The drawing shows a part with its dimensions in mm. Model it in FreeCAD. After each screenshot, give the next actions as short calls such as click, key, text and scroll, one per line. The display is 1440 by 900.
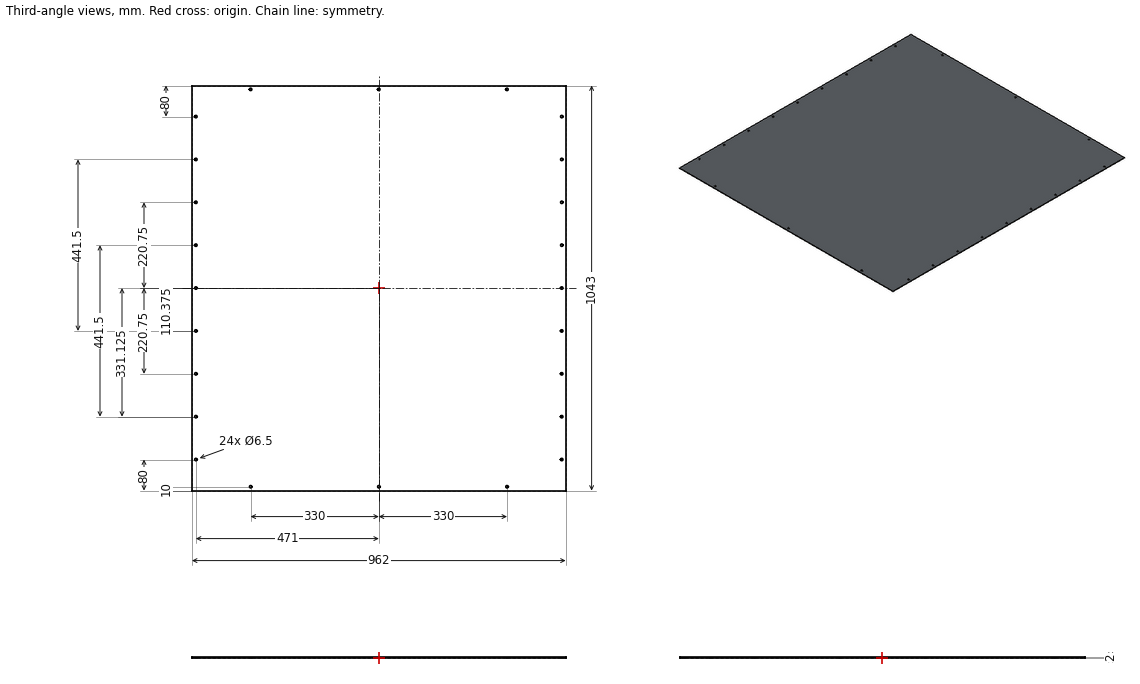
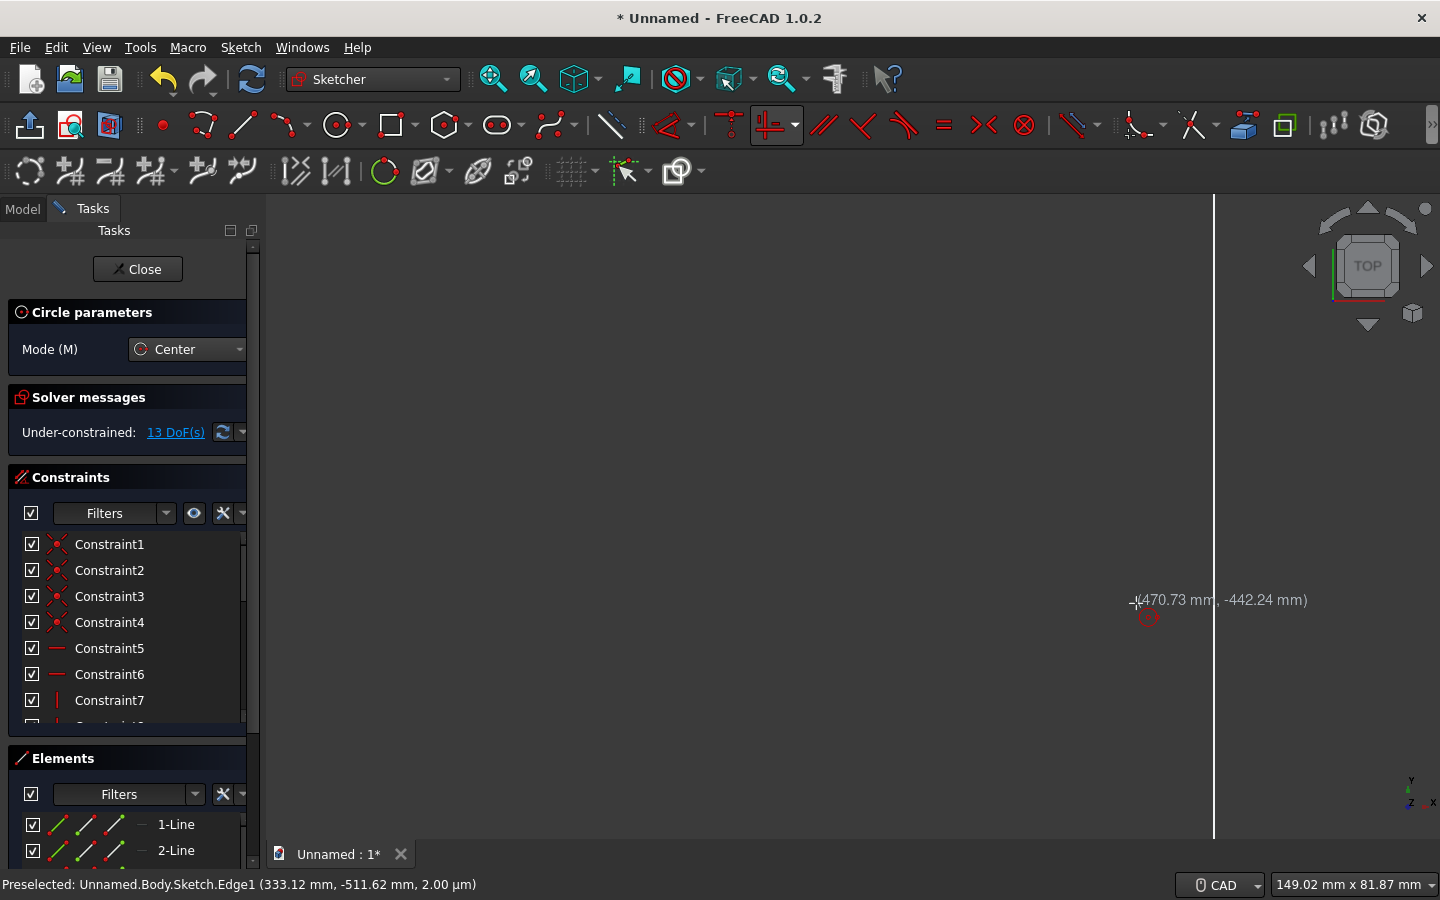
scroll(961, 694, down, 15)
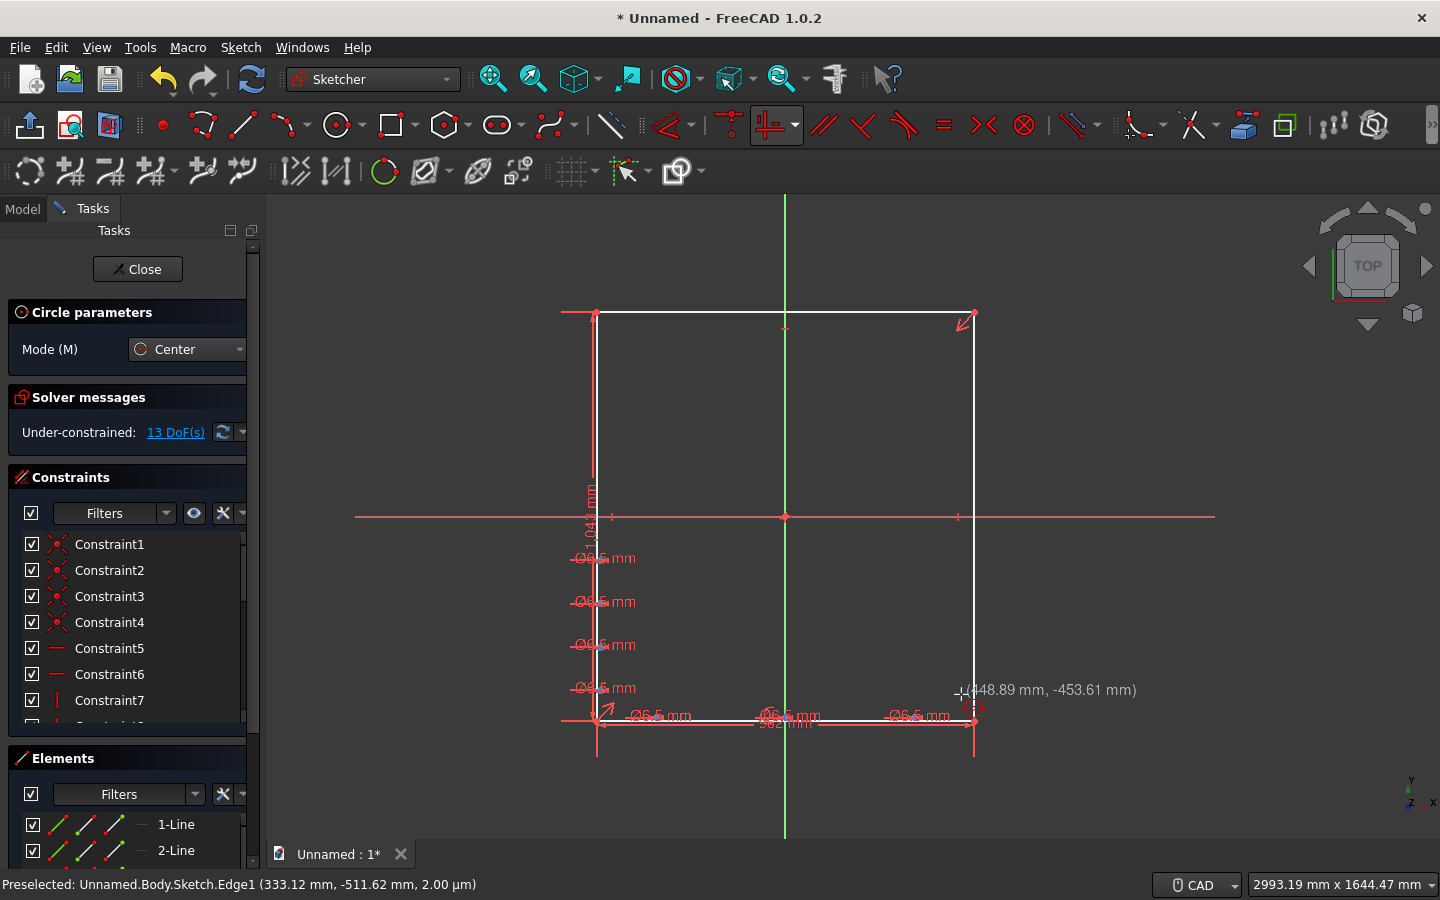
scroll(970, 690, up, 7)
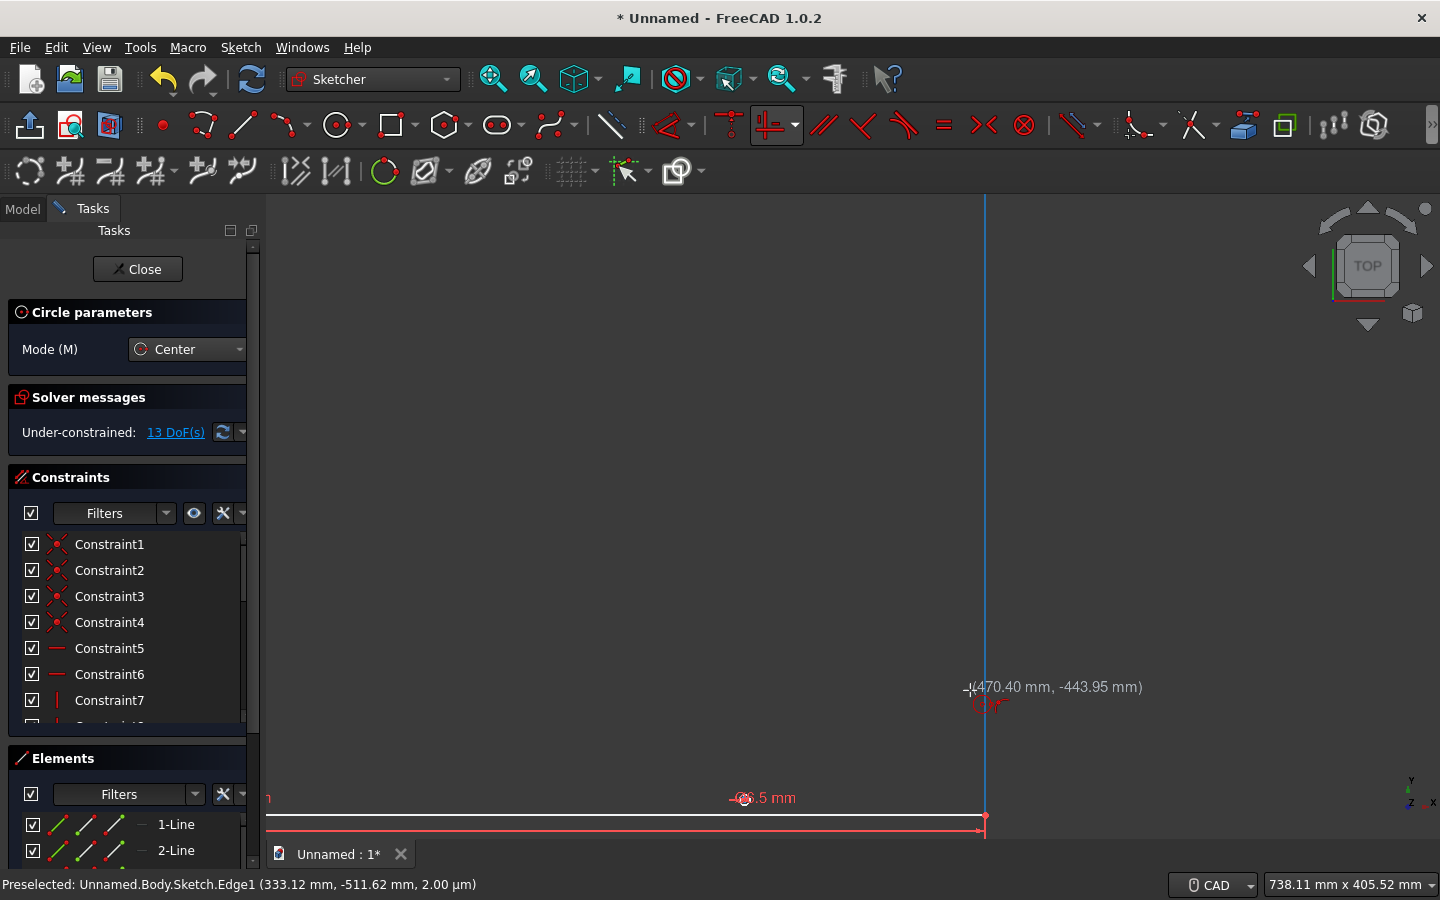
click(969, 688)
move(965, 684)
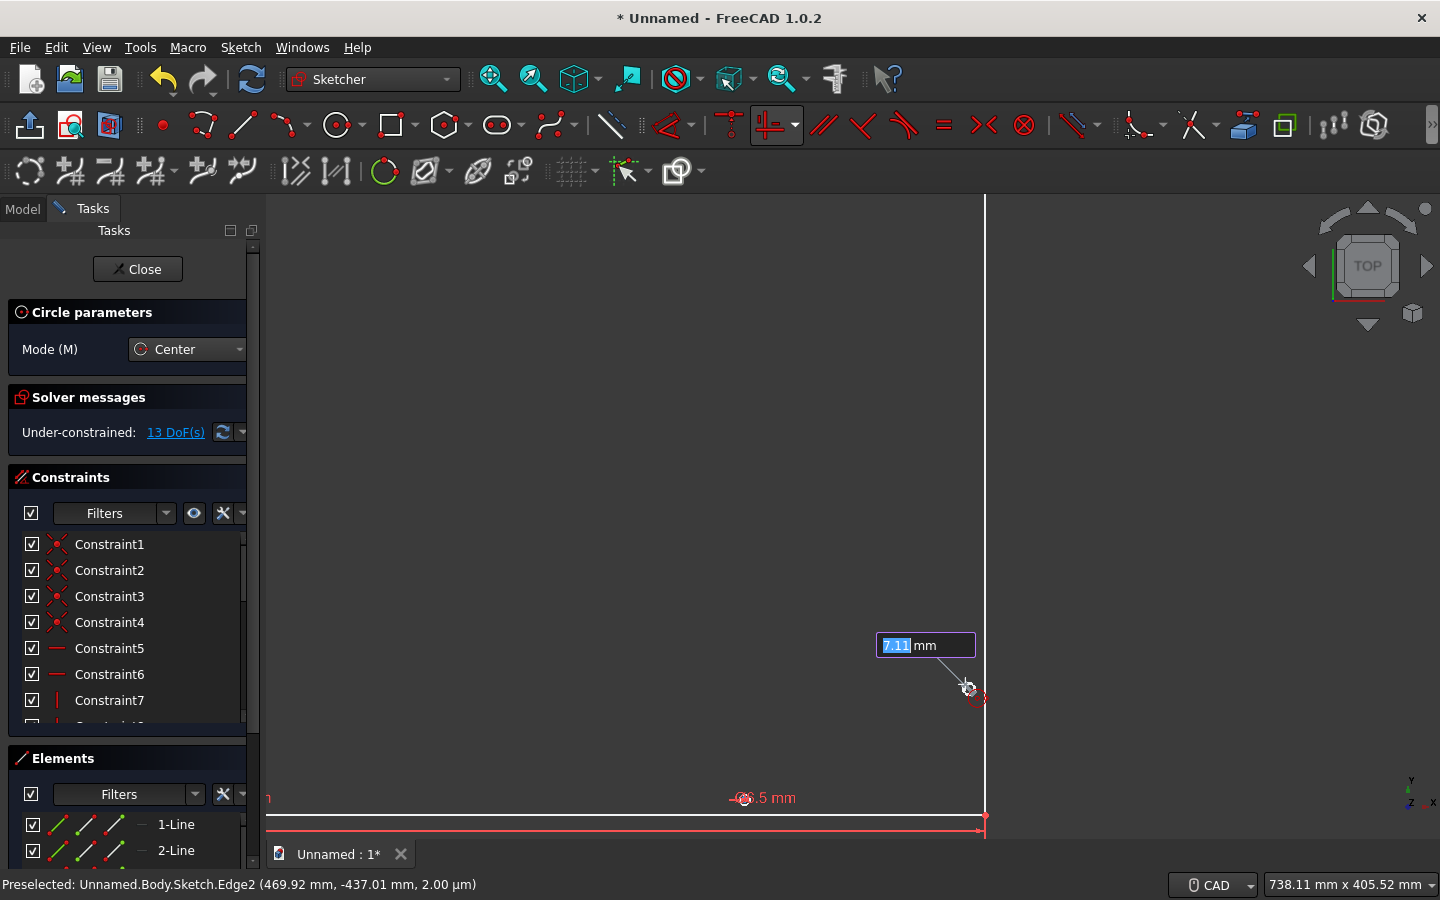
text(6.5)
key(Return)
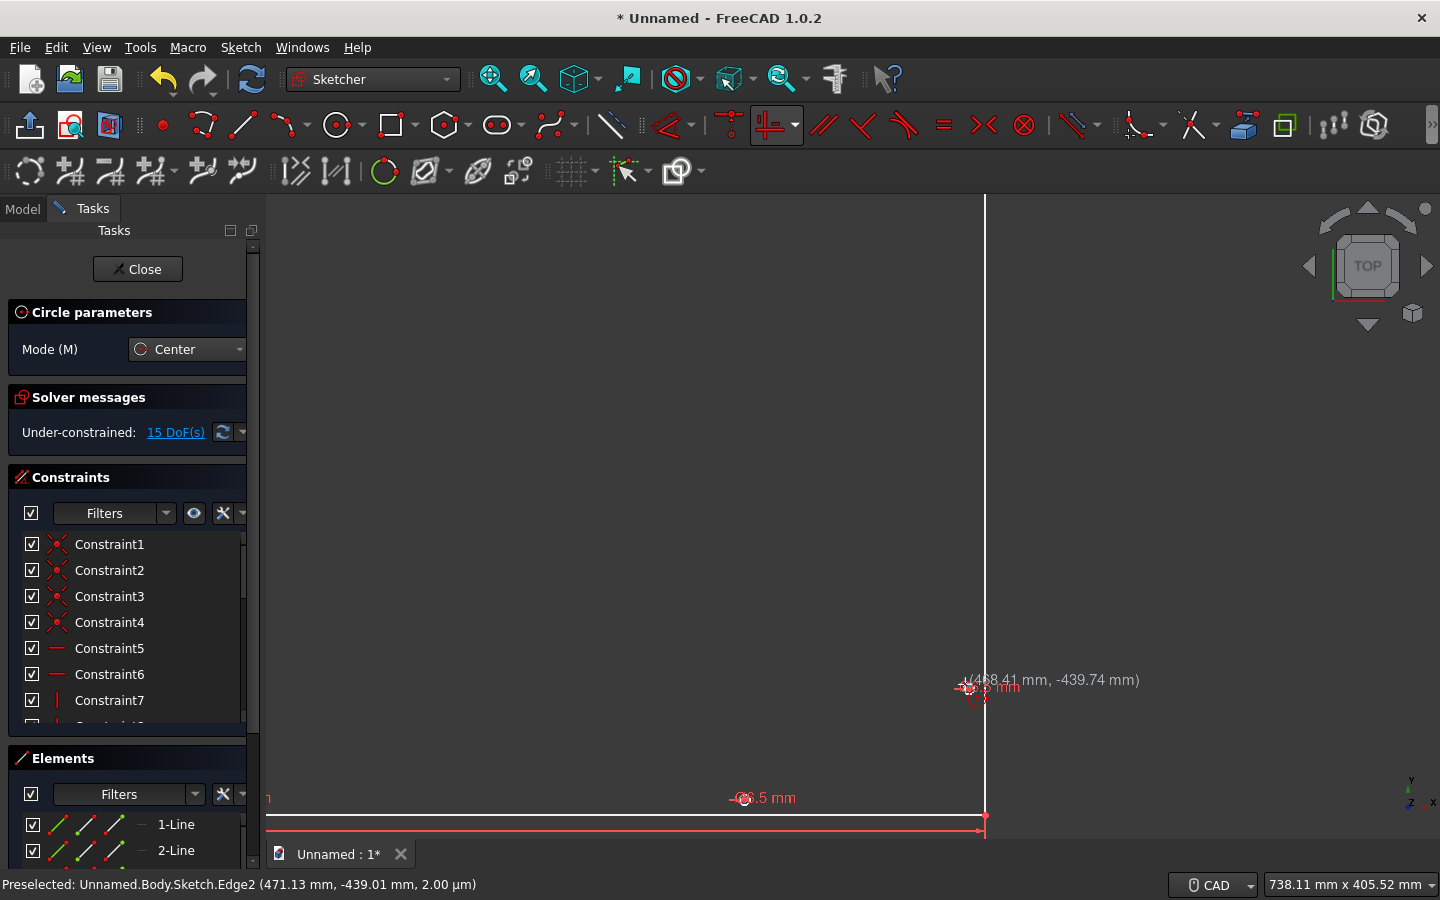
scroll(969, 512, up, 8)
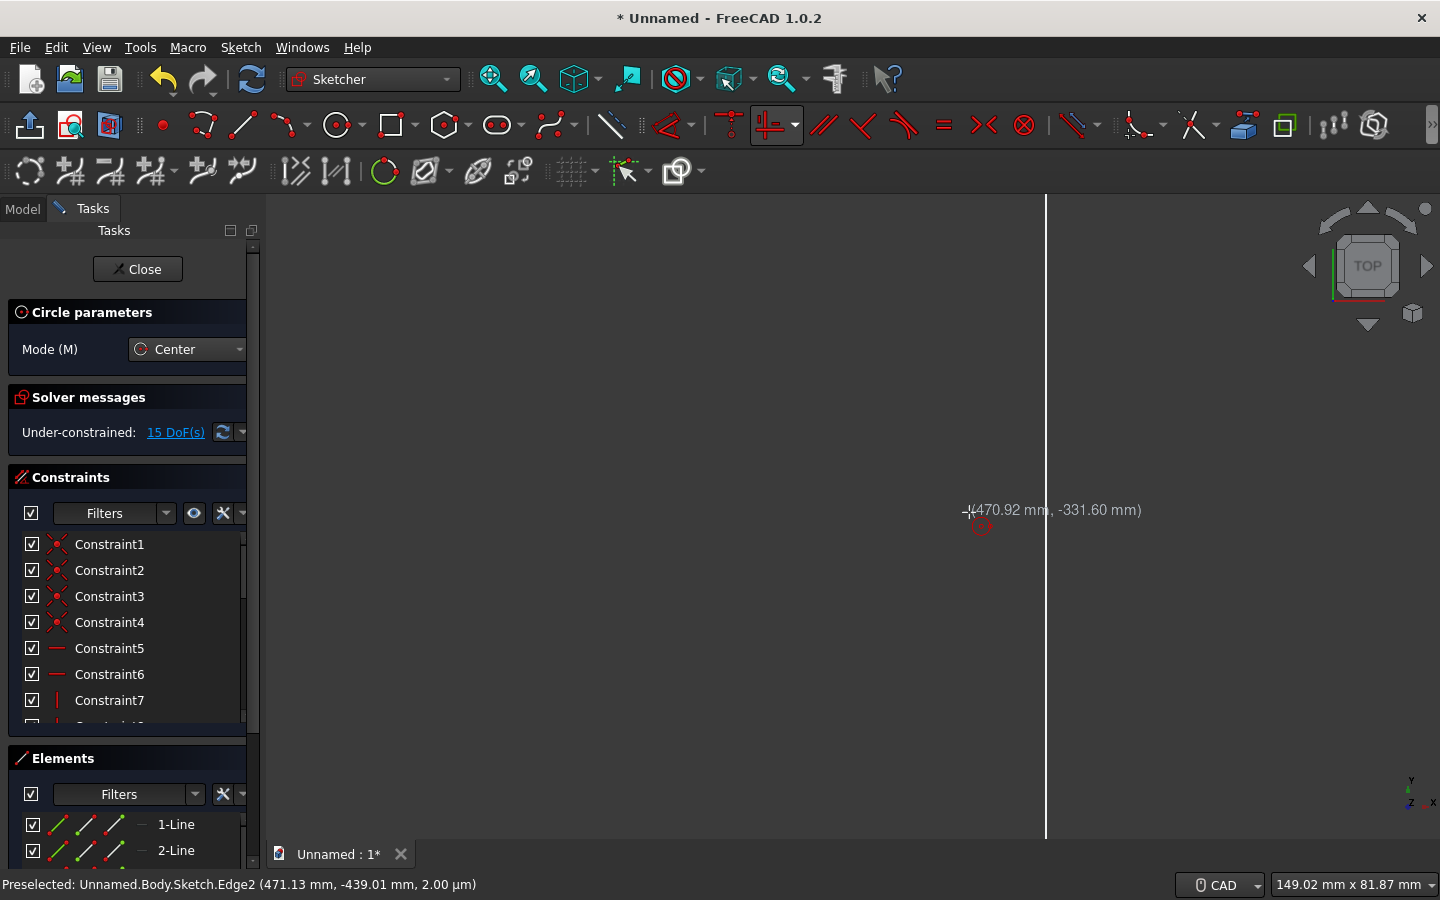
scroll(969, 653, down, 15)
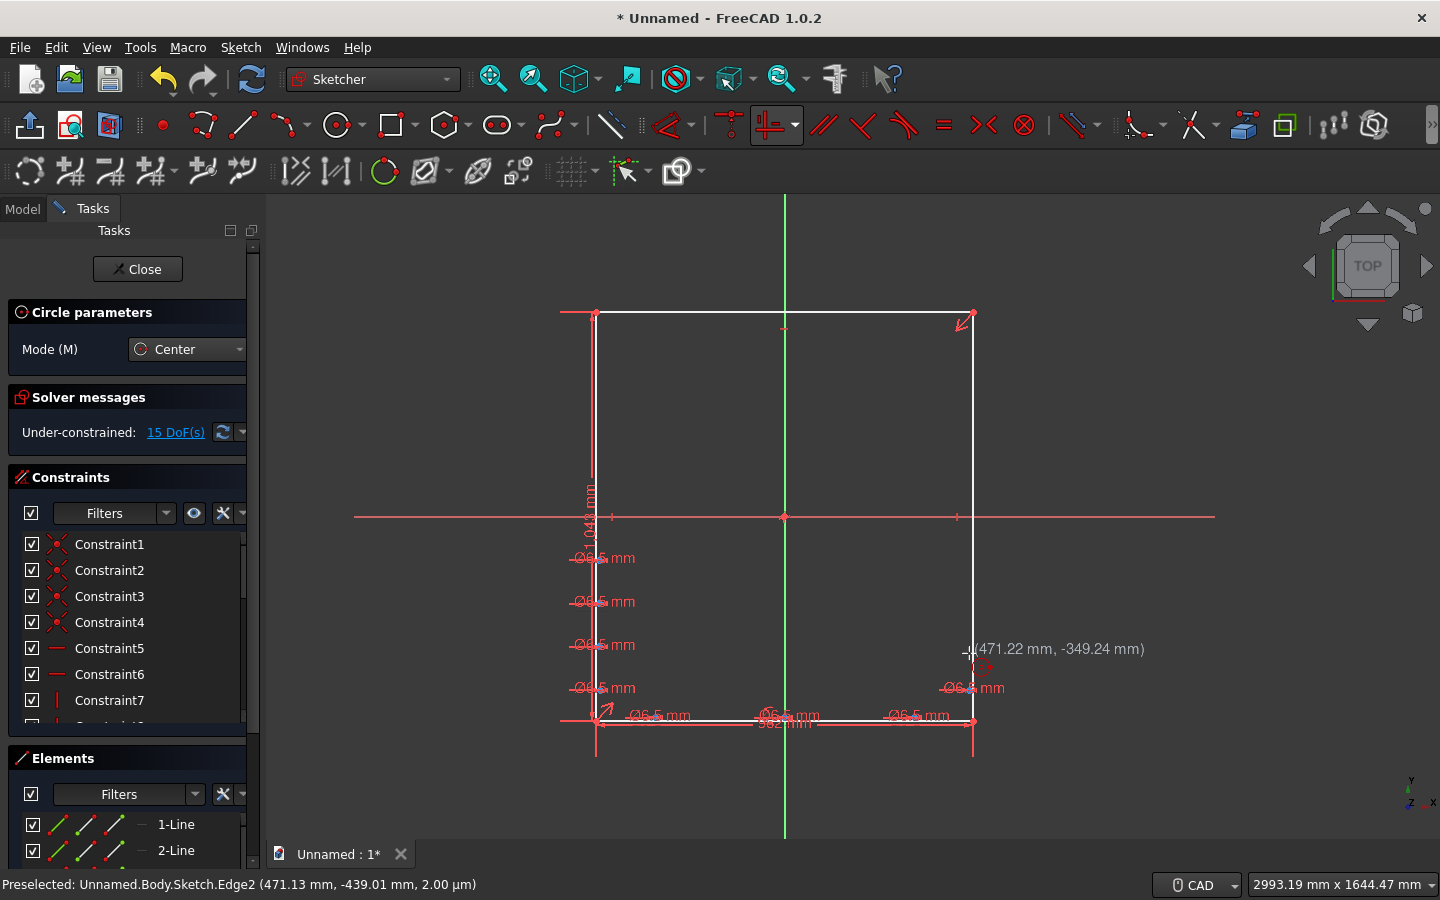
scroll(969, 647, up, 7)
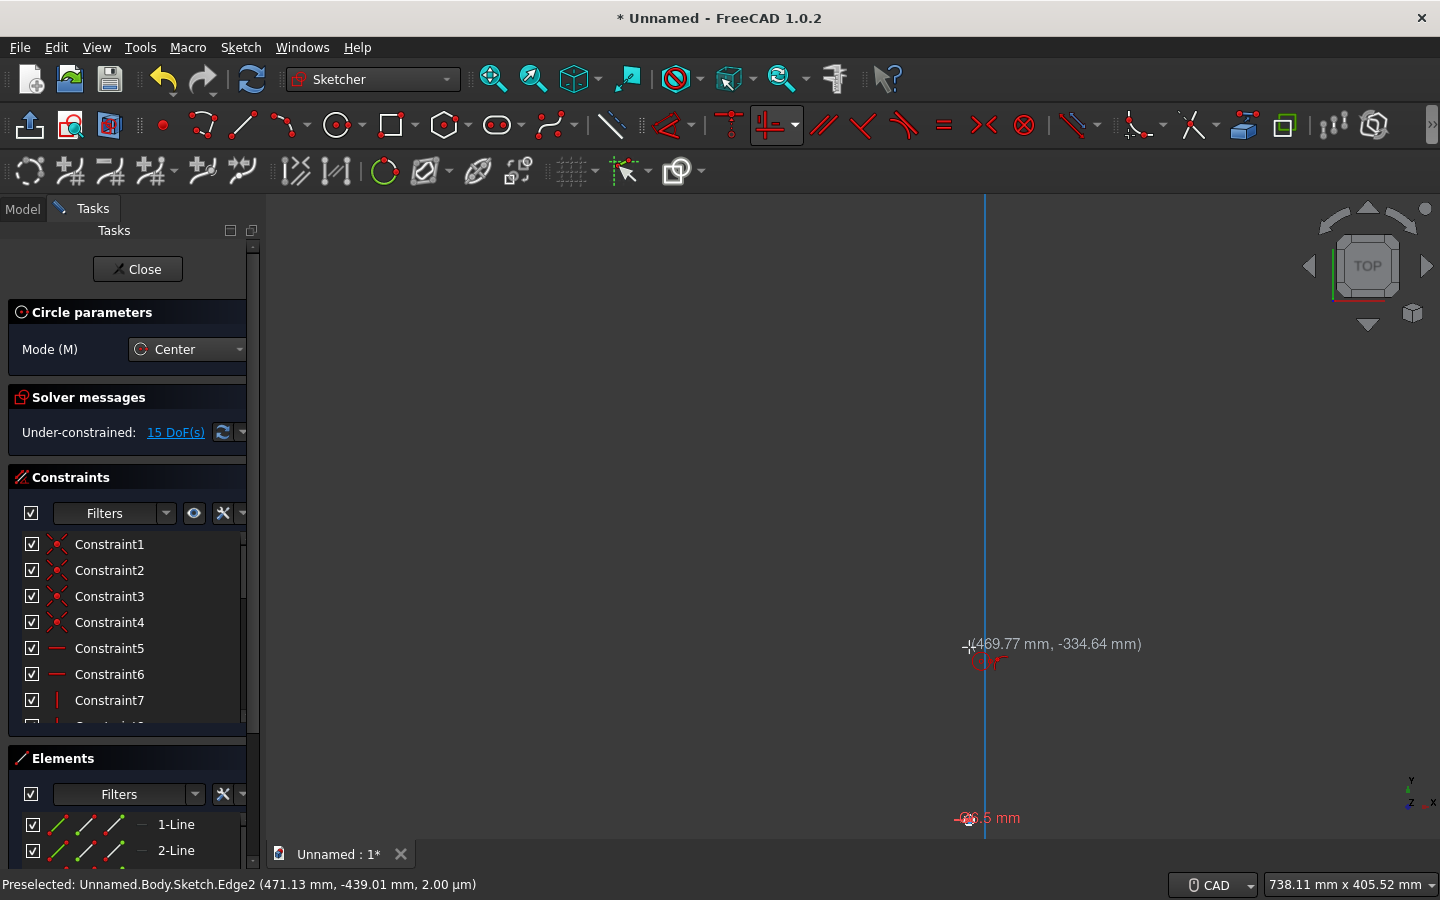
click(969, 643)
move(965, 640)